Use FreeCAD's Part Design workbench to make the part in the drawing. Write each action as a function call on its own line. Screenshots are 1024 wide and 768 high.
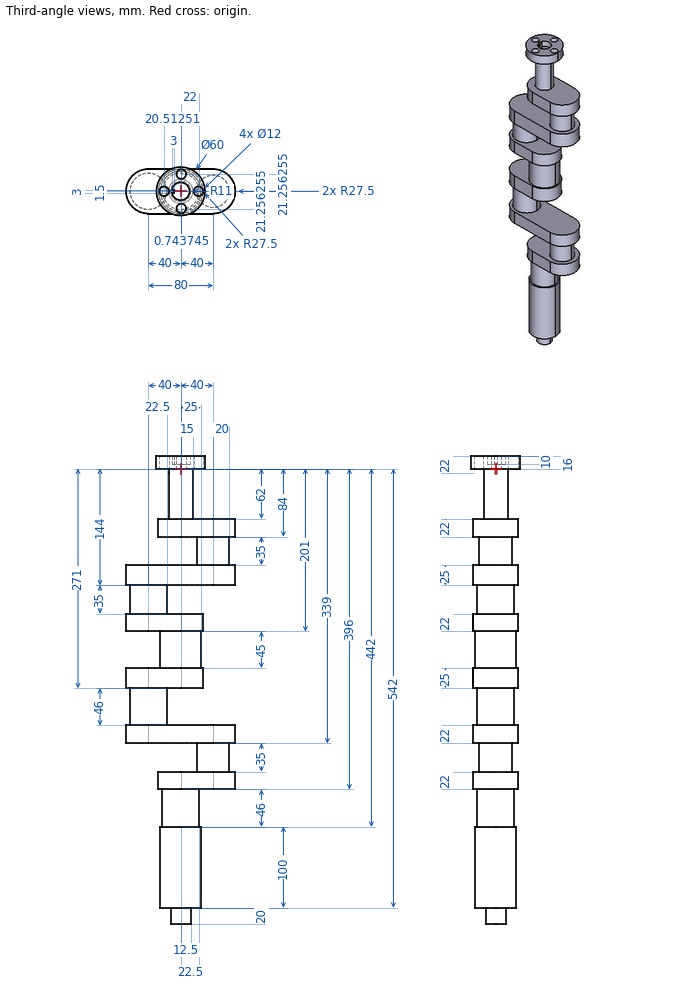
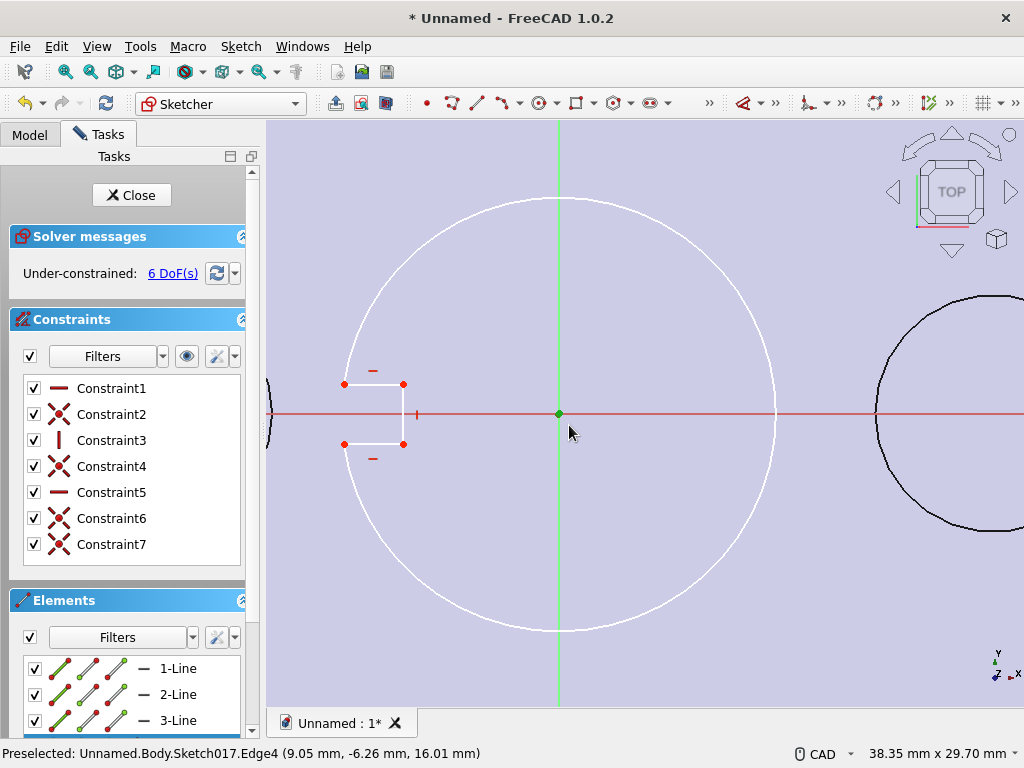
key(c)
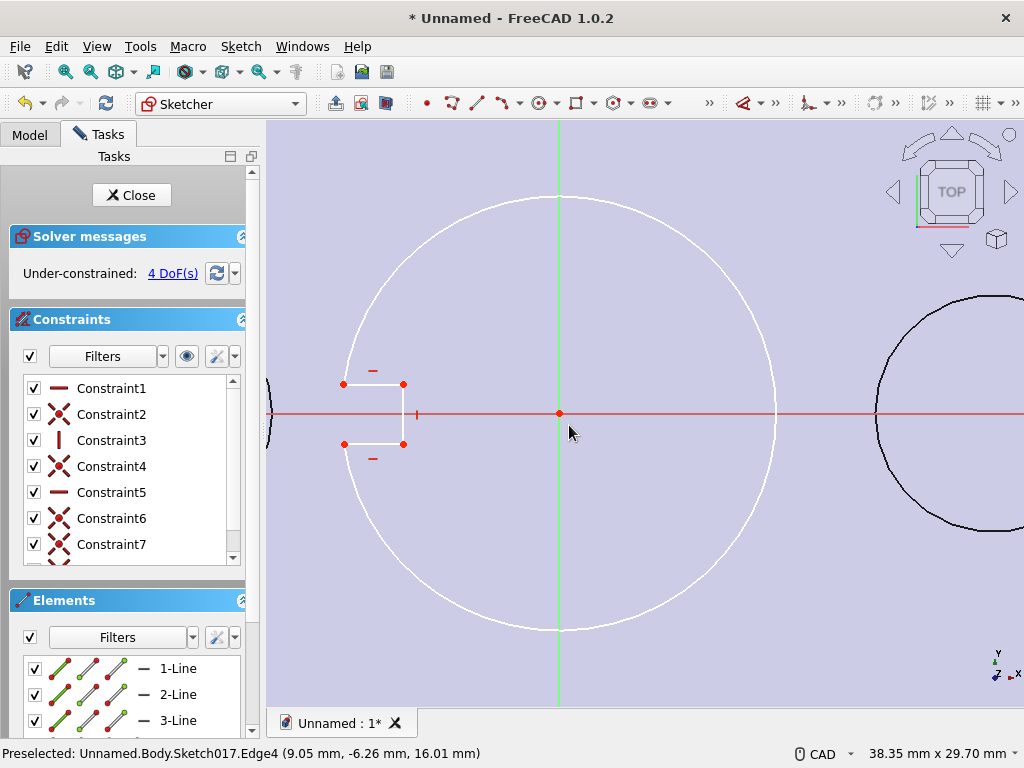
key(d)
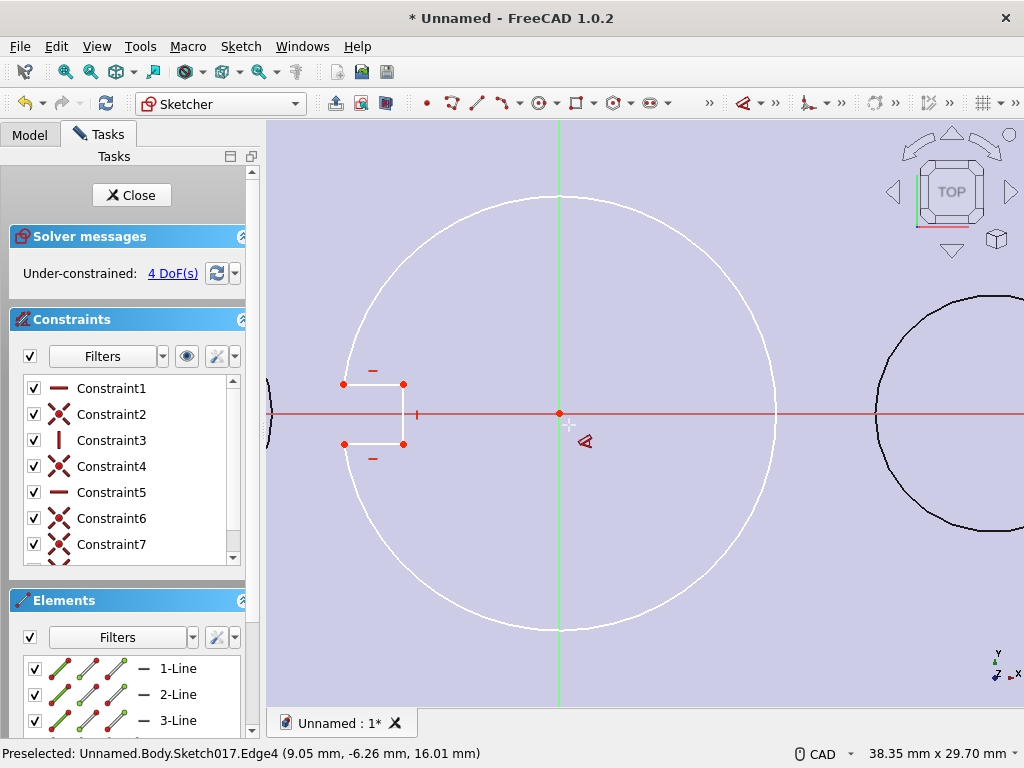
click(638, 616)
click(650, 646)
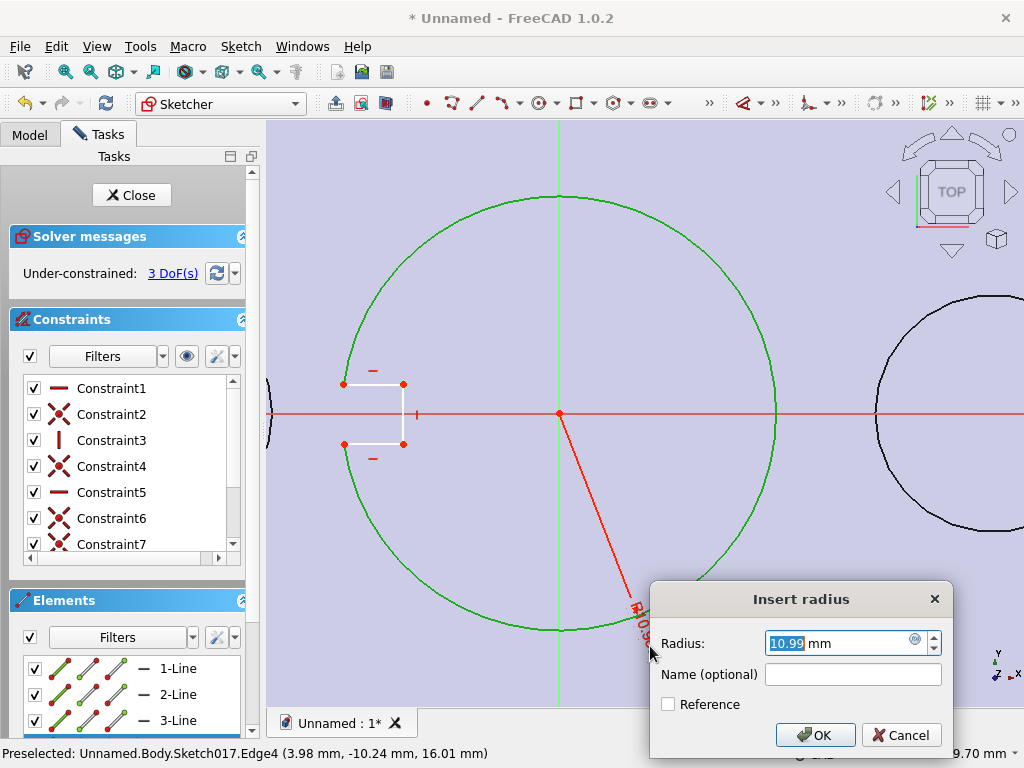
text(11)
key(Return)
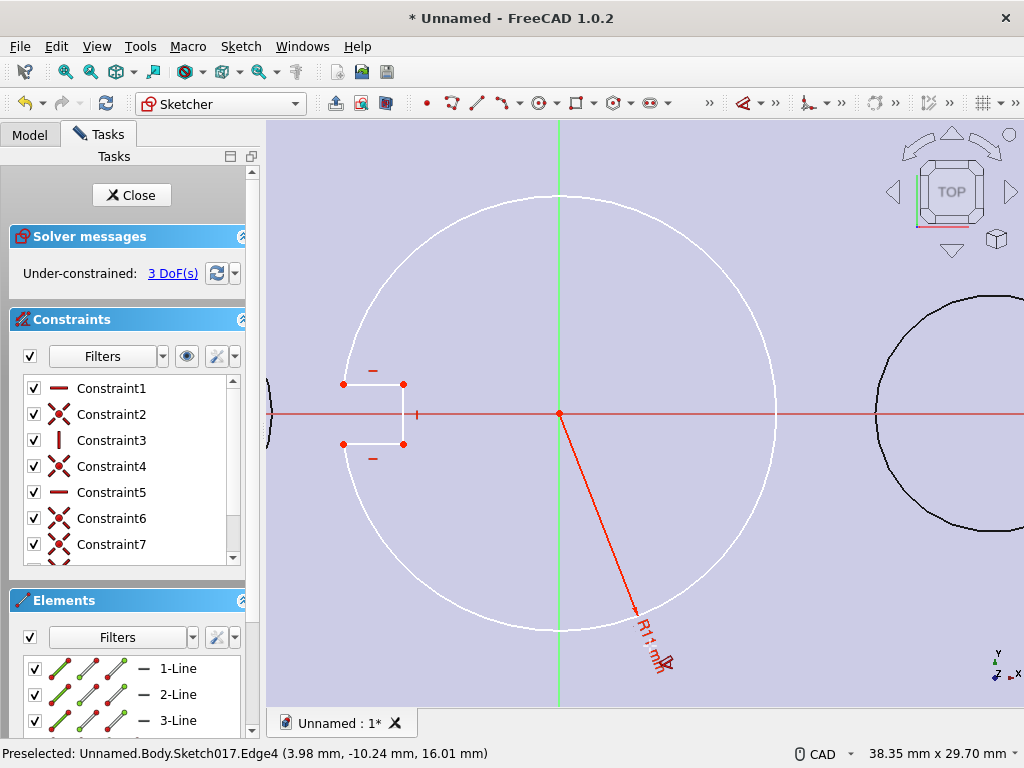
click(361, 385)
click(373, 351)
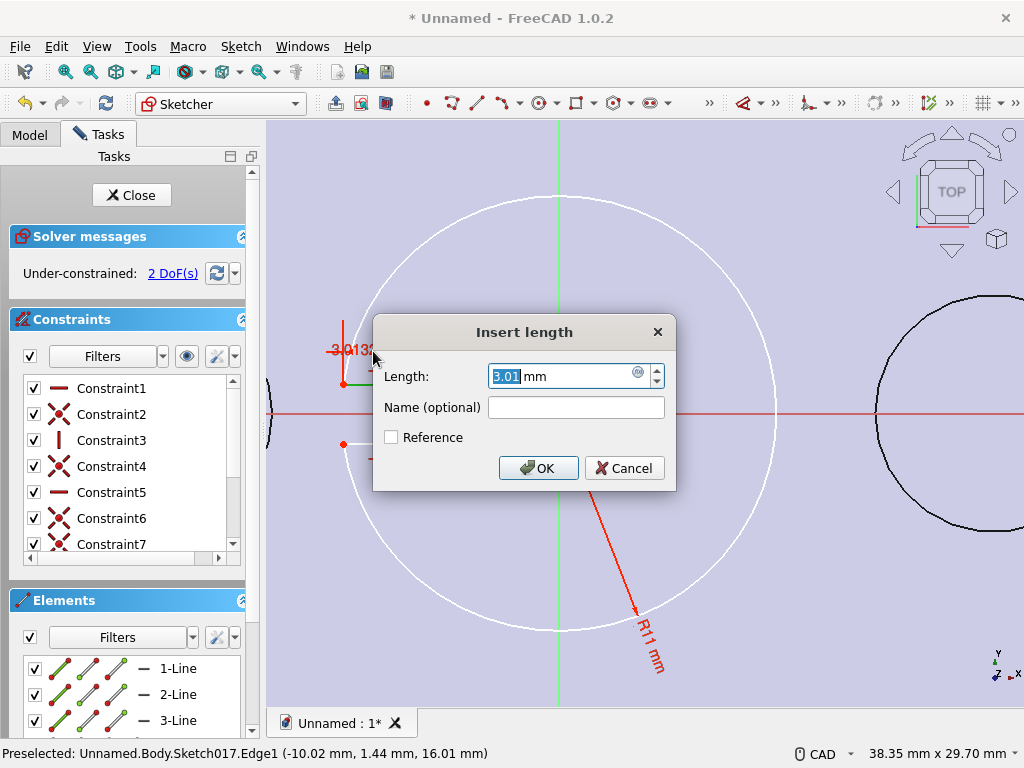
text(3)
key(Return)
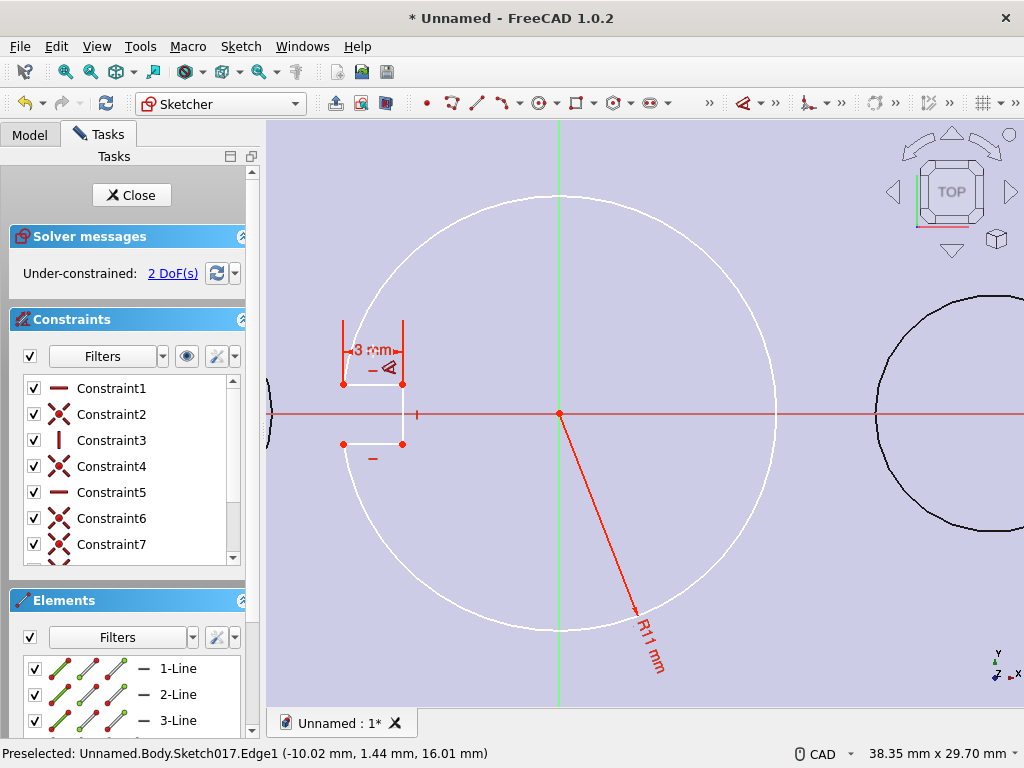
scroll(403, 403, up, 2)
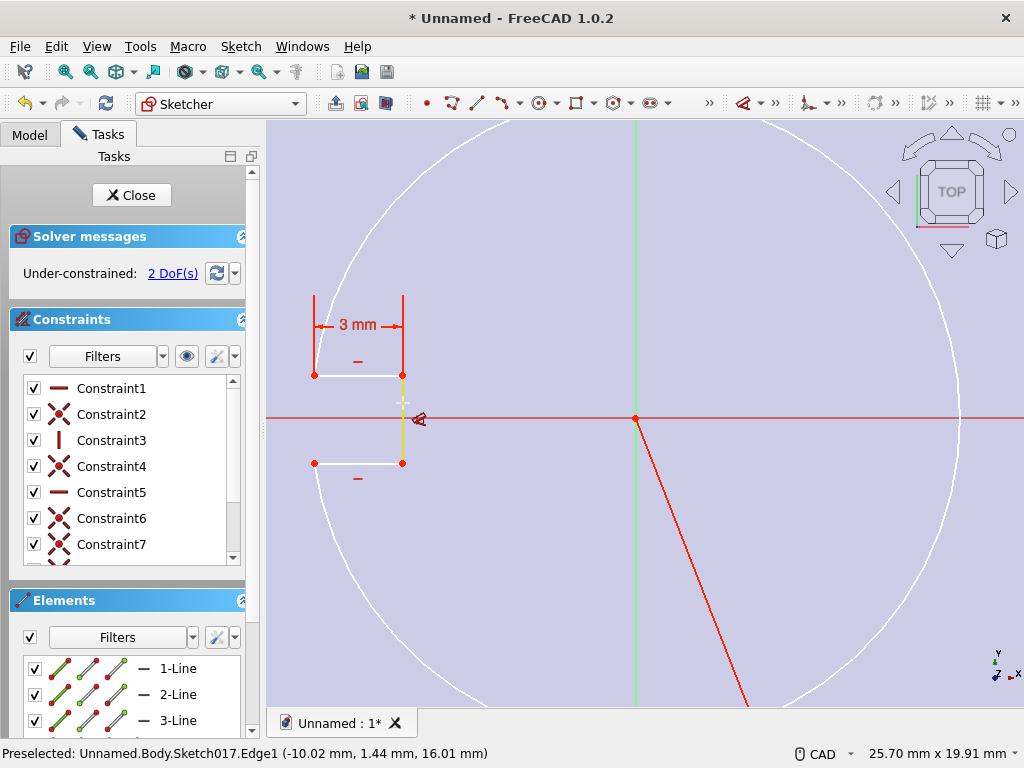
click(403, 402)
click(369, 400)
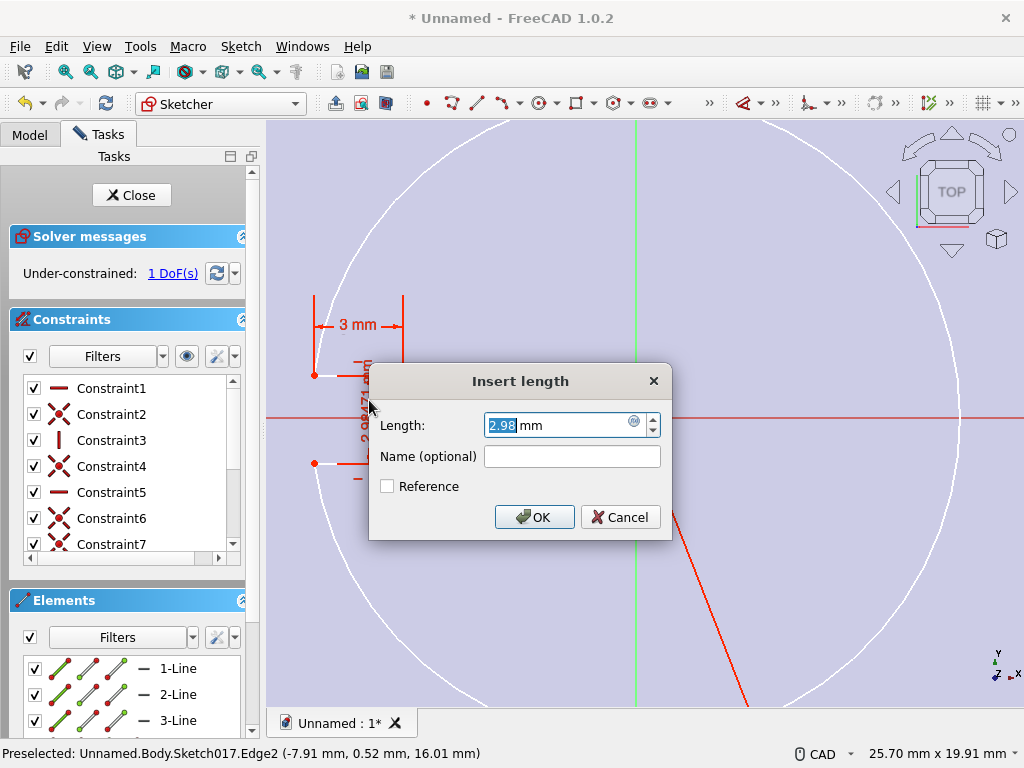
text(3)
key(Return)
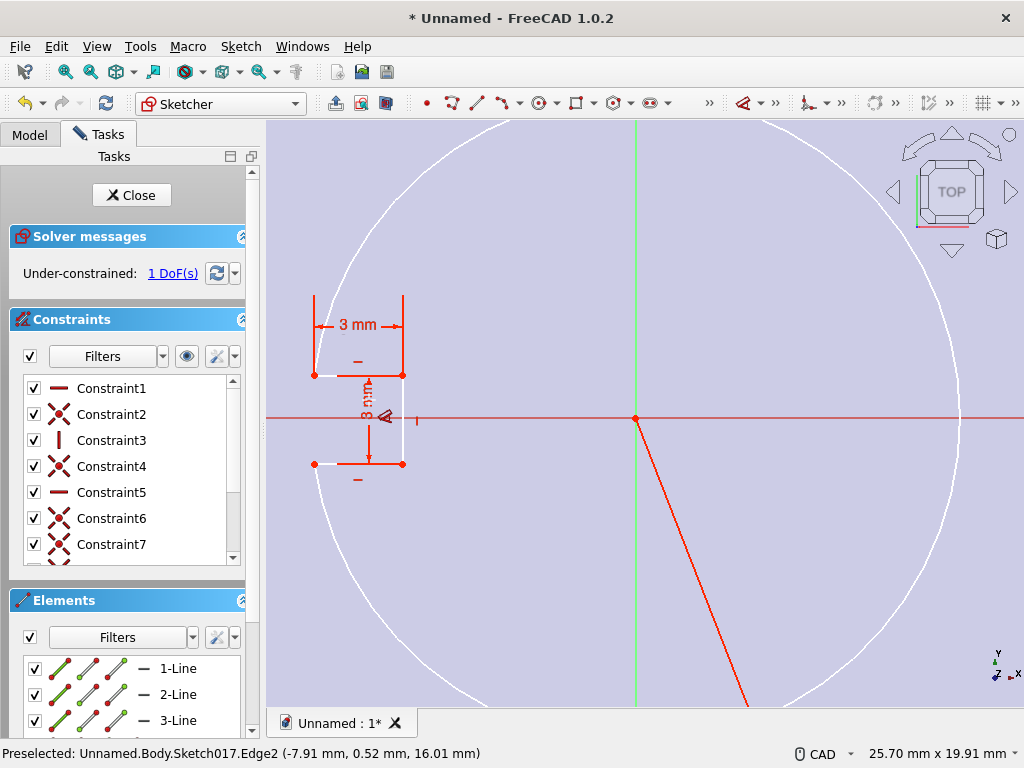
click(314, 376)
click(670, 397)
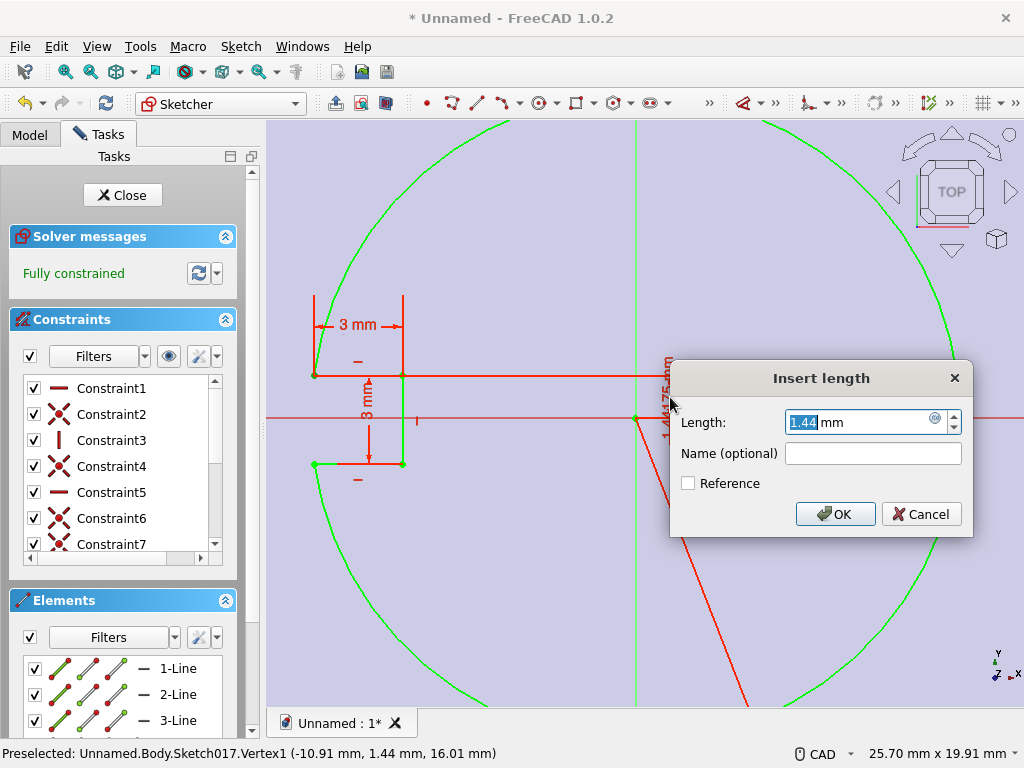
text(1.5)
key(Return)
key(Escape)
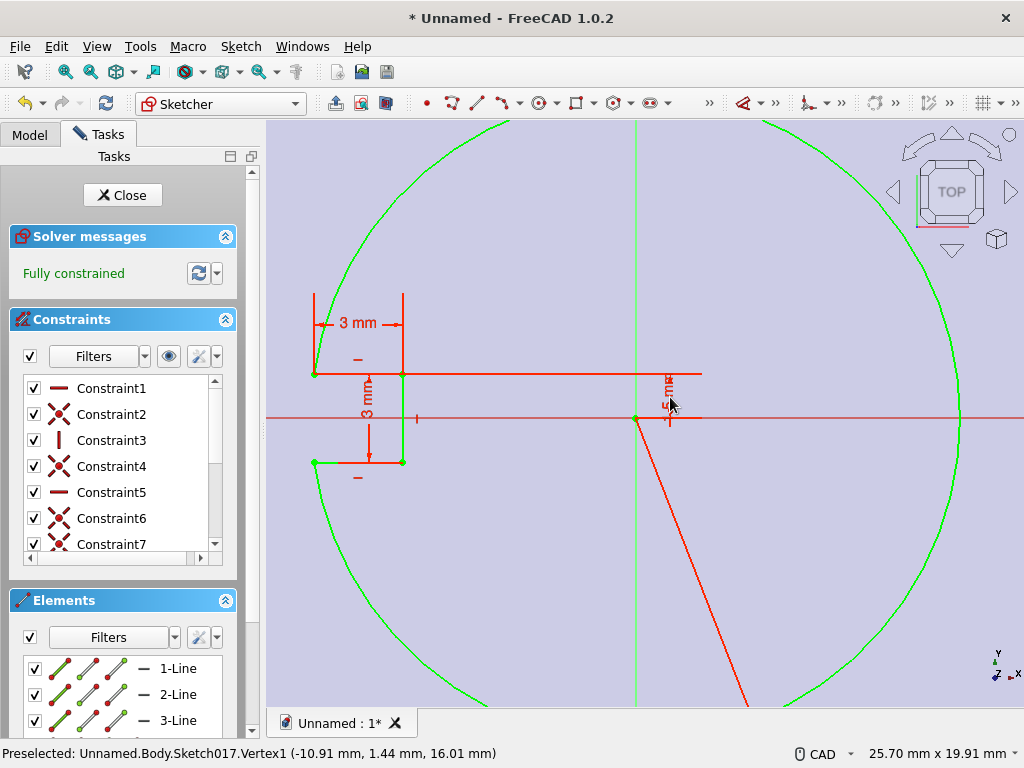
click(123, 195)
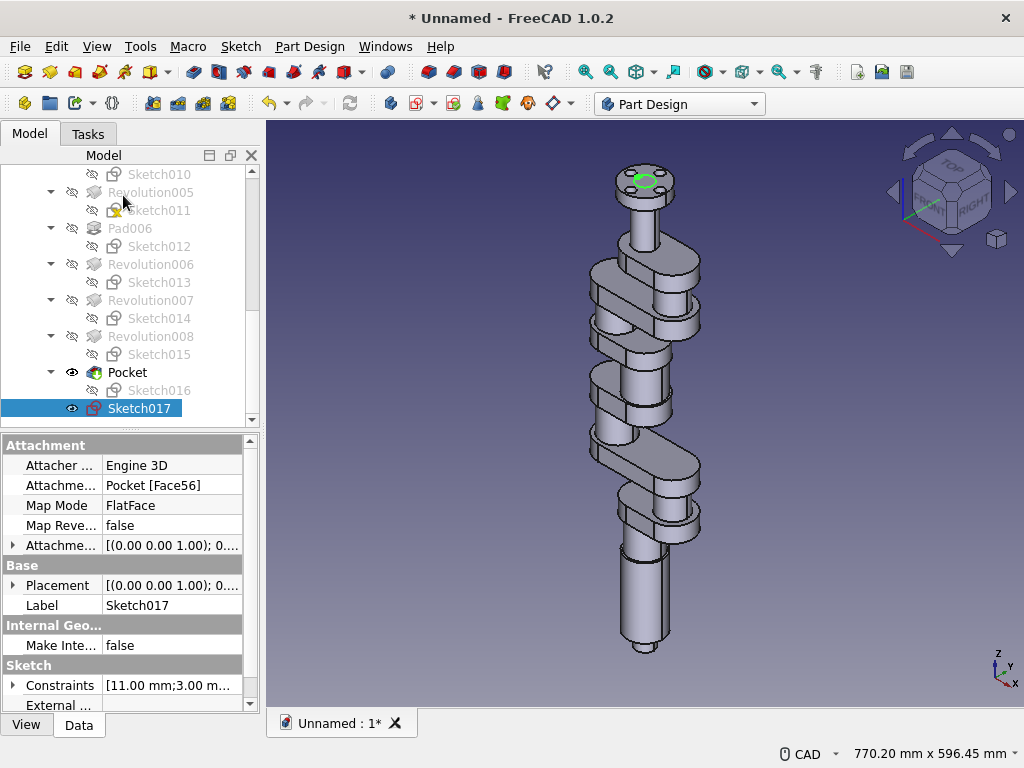
click(194, 72)